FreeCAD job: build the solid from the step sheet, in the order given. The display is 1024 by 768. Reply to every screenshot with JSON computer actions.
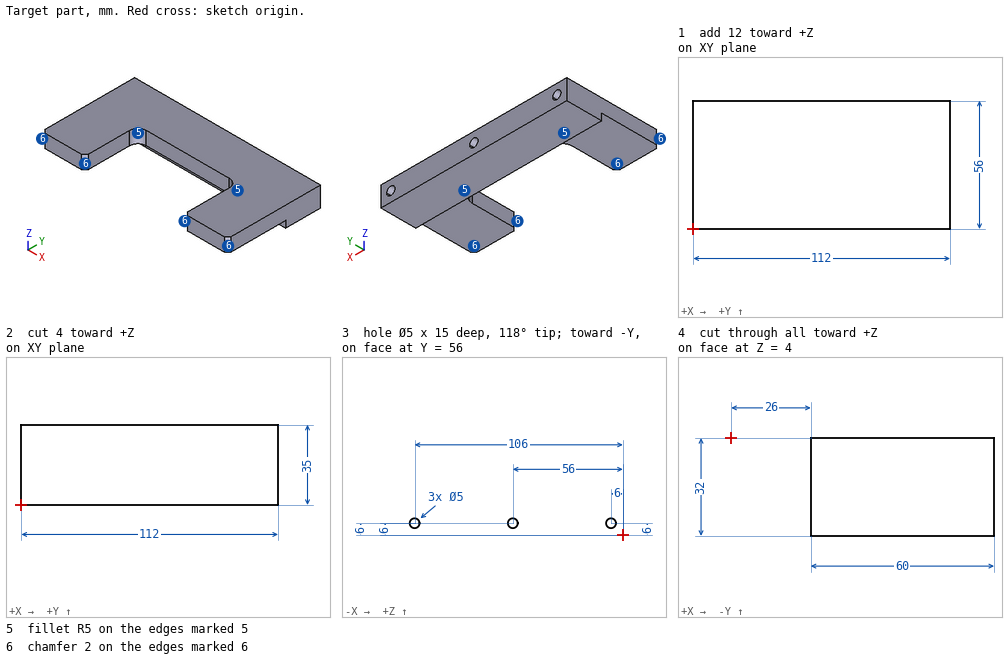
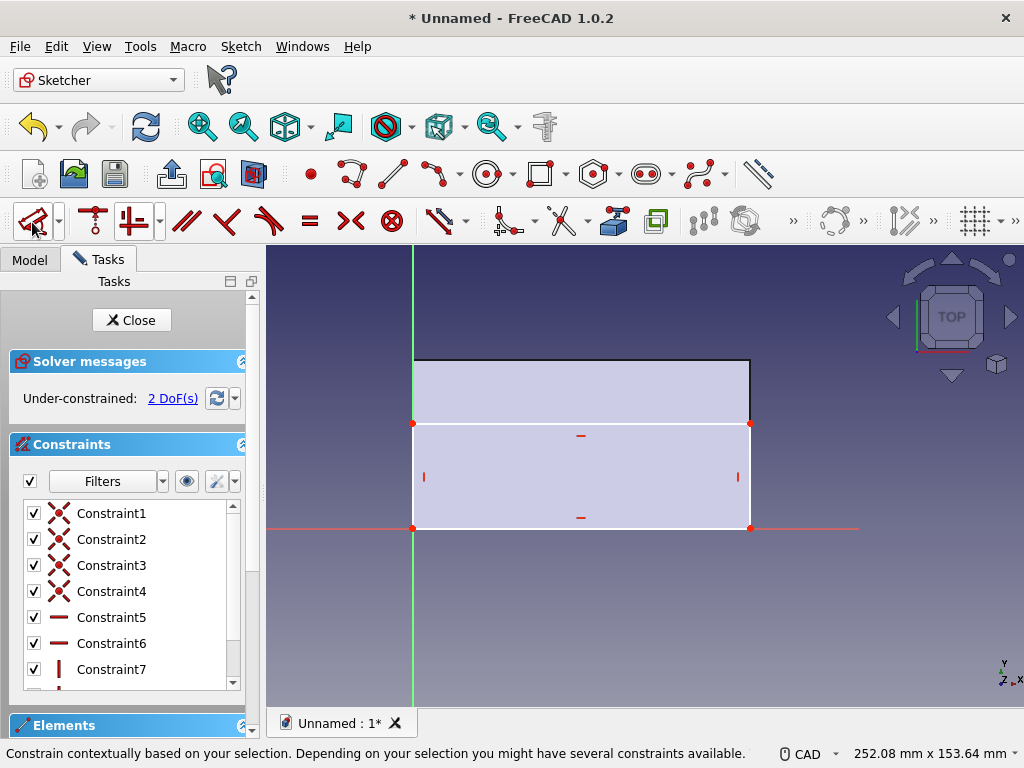
{"action": "left_click", "coordinate": [750, 497]}
{"action": "left_click", "coordinate": [784, 476]}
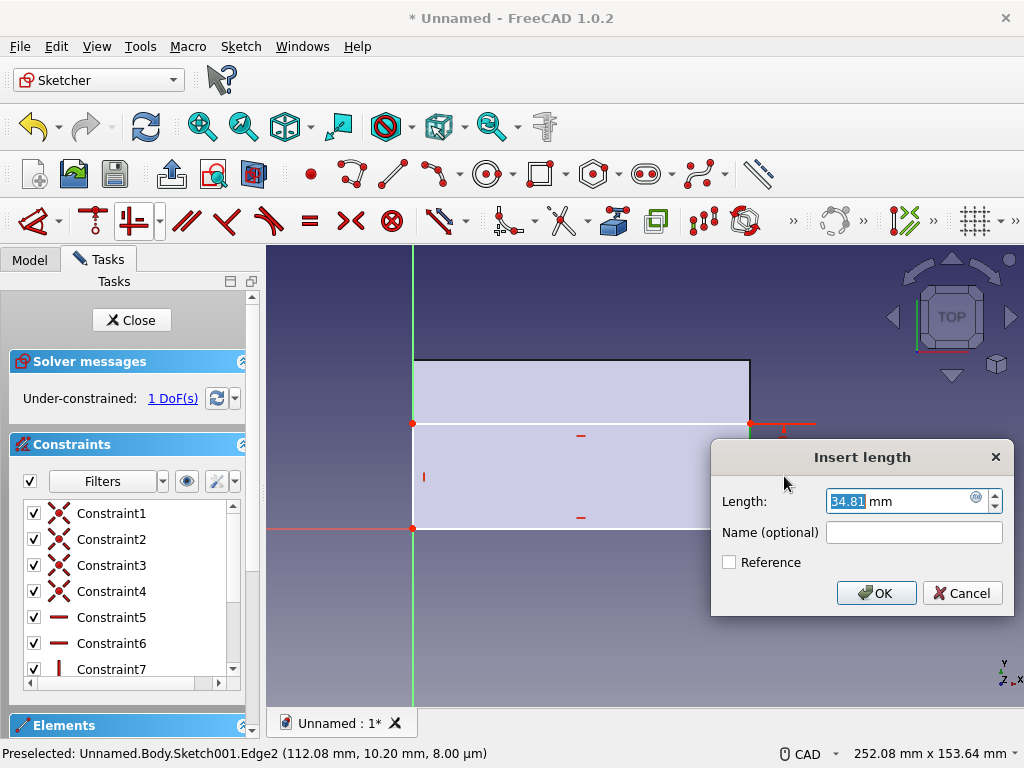
{"action": "type", "text": "35"}
{"action": "key", "text": "Return"}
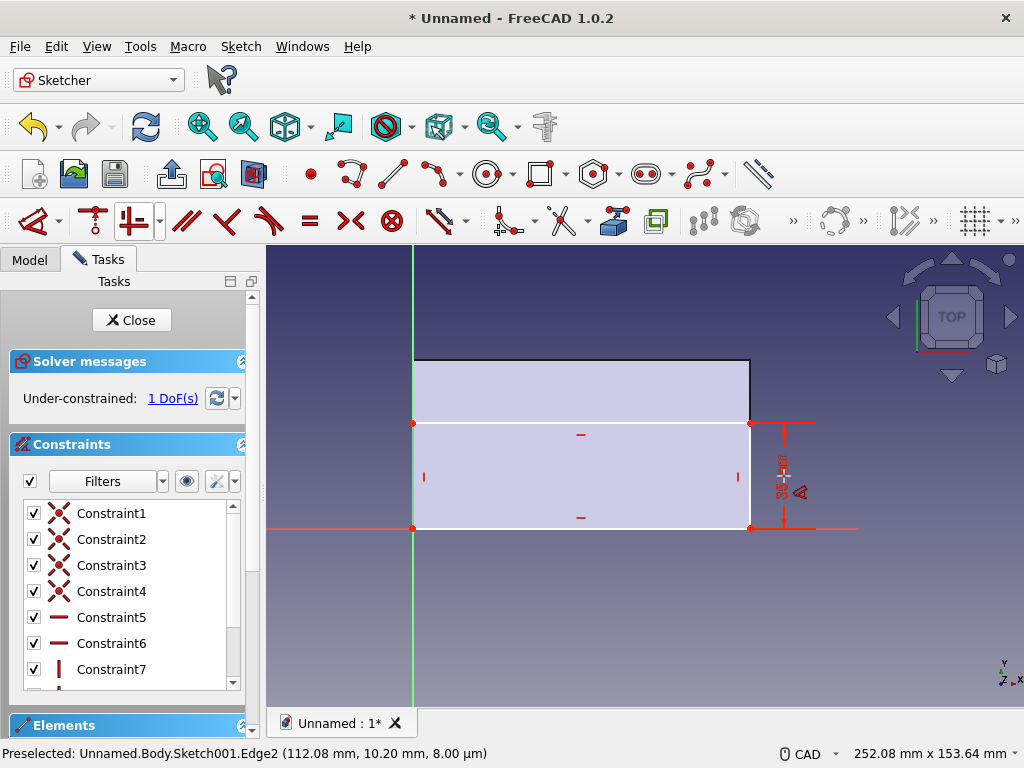
{"action": "left_click", "coordinate": [514, 529]}
{"action": "left_click", "coordinate": [581, 563]}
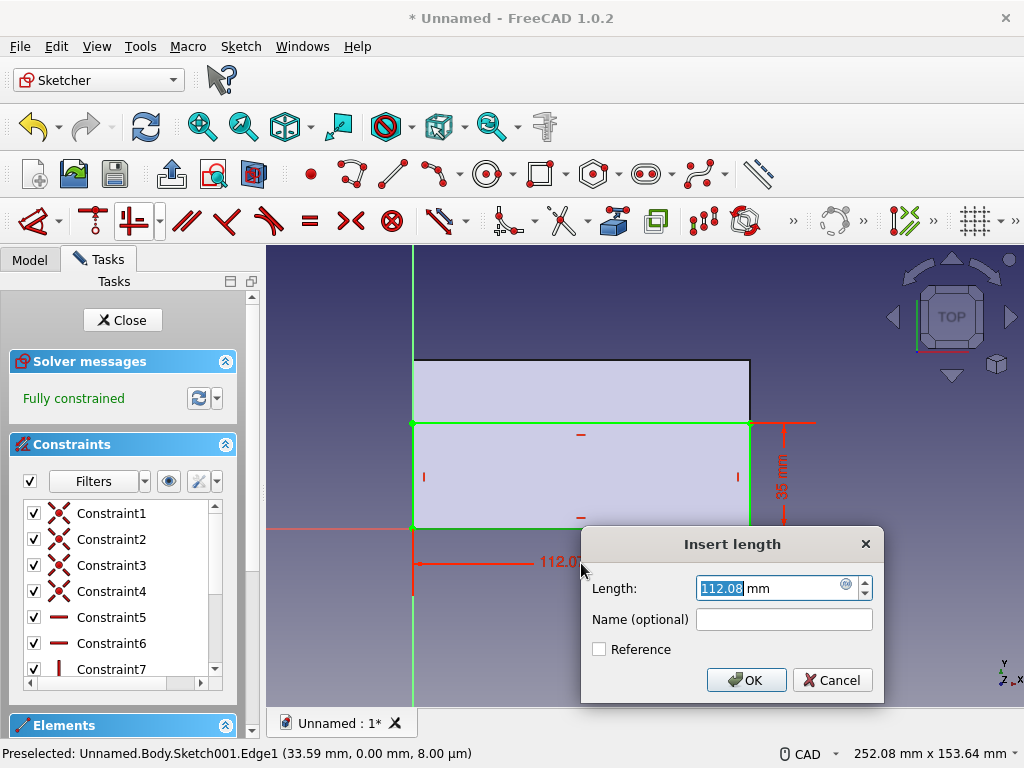
{"action": "type", "text": "112"}
{"action": "key", "text": "Return"}
{"action": "key", "text": "Escape"}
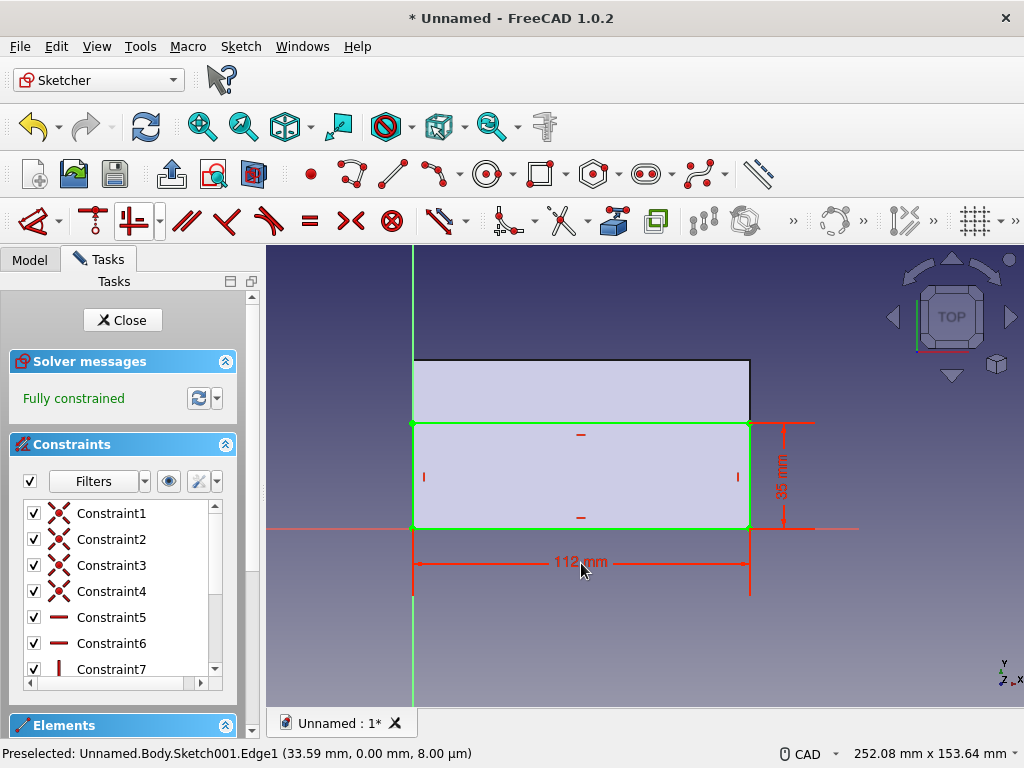
{"action": "left_click", "coordinate": [123, 320]}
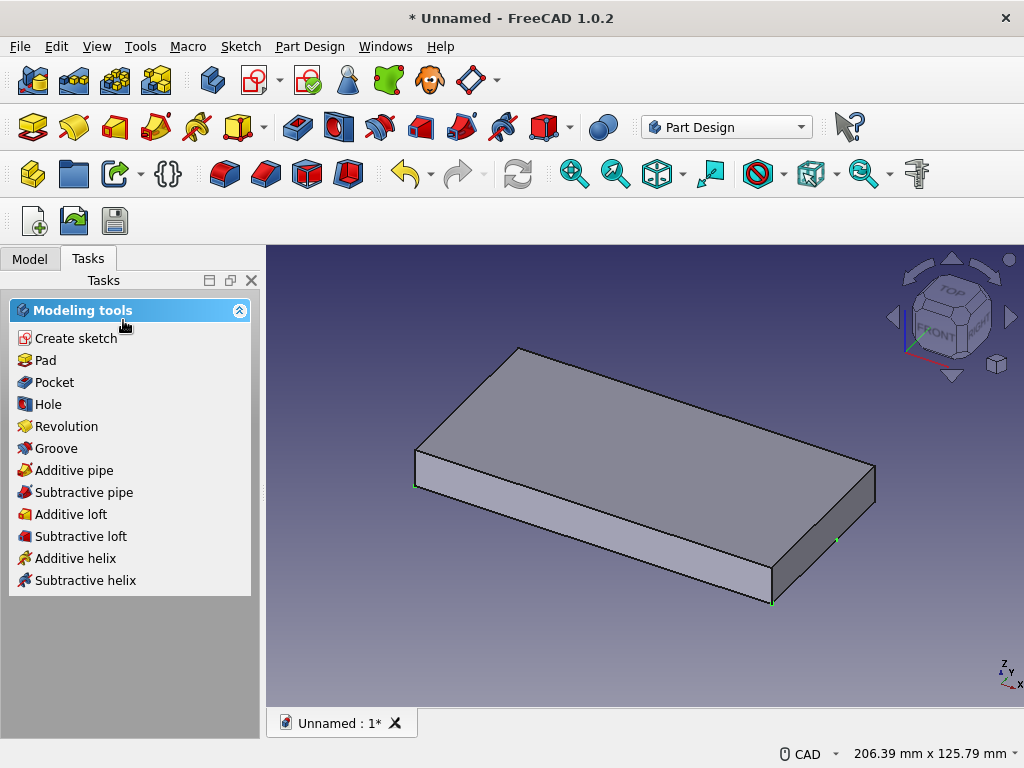
{"action": "left_click", "coordinate": [298, 128]}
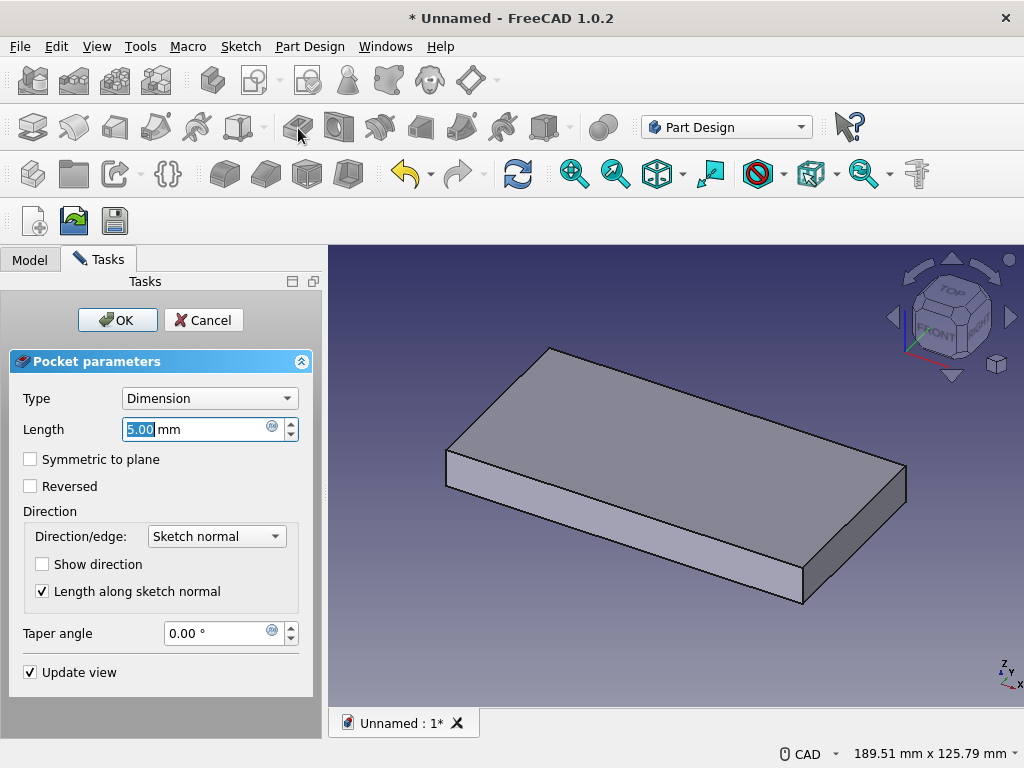
{"action": "type", "text": "4"}
{"action": "key", "text": "Tab"}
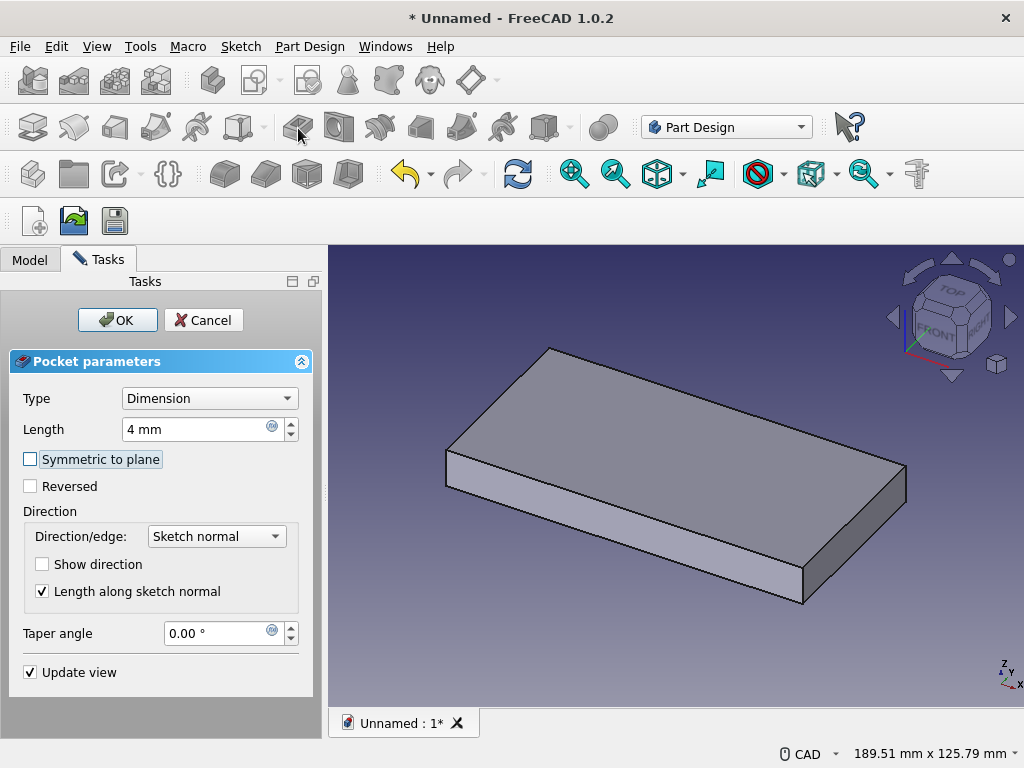
{"action": "left_click", "coordinate": [31, 486]}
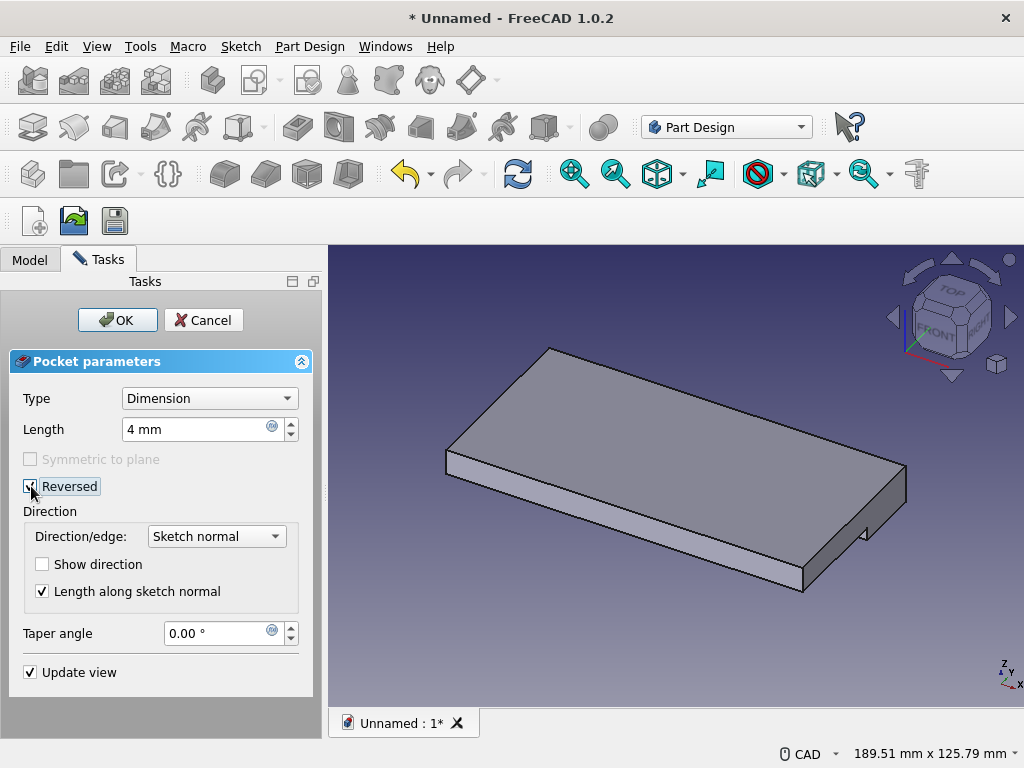
{"action": "left_click", "coordinate": [118, 320]}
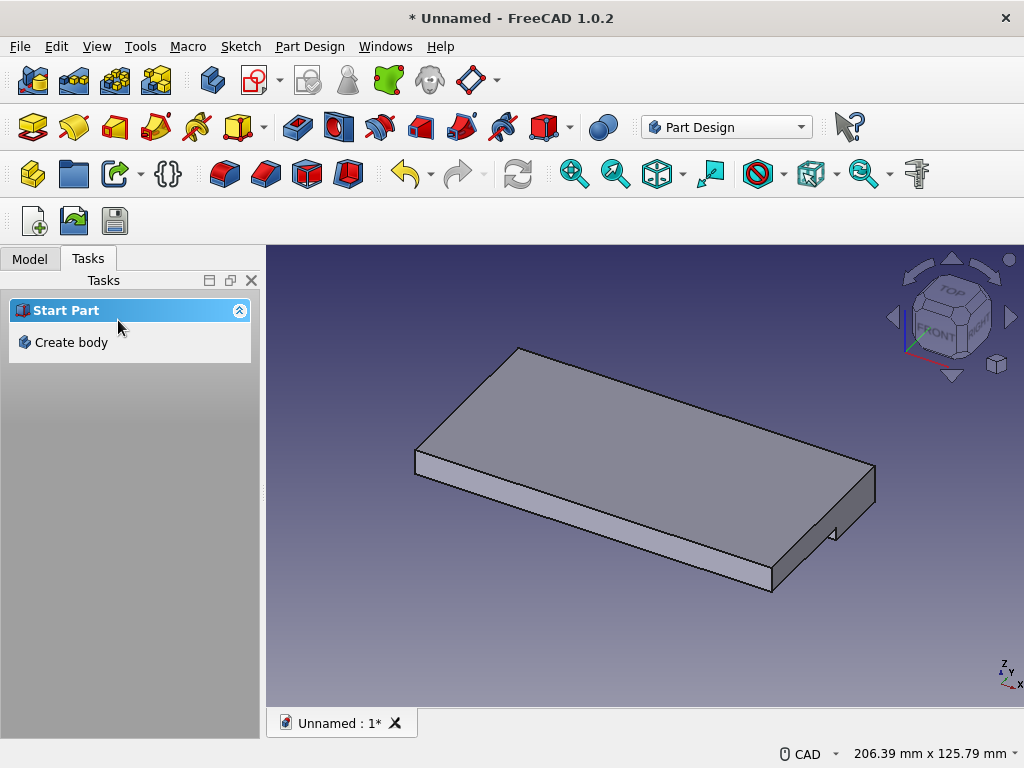
{"action": "key", "text": "4"}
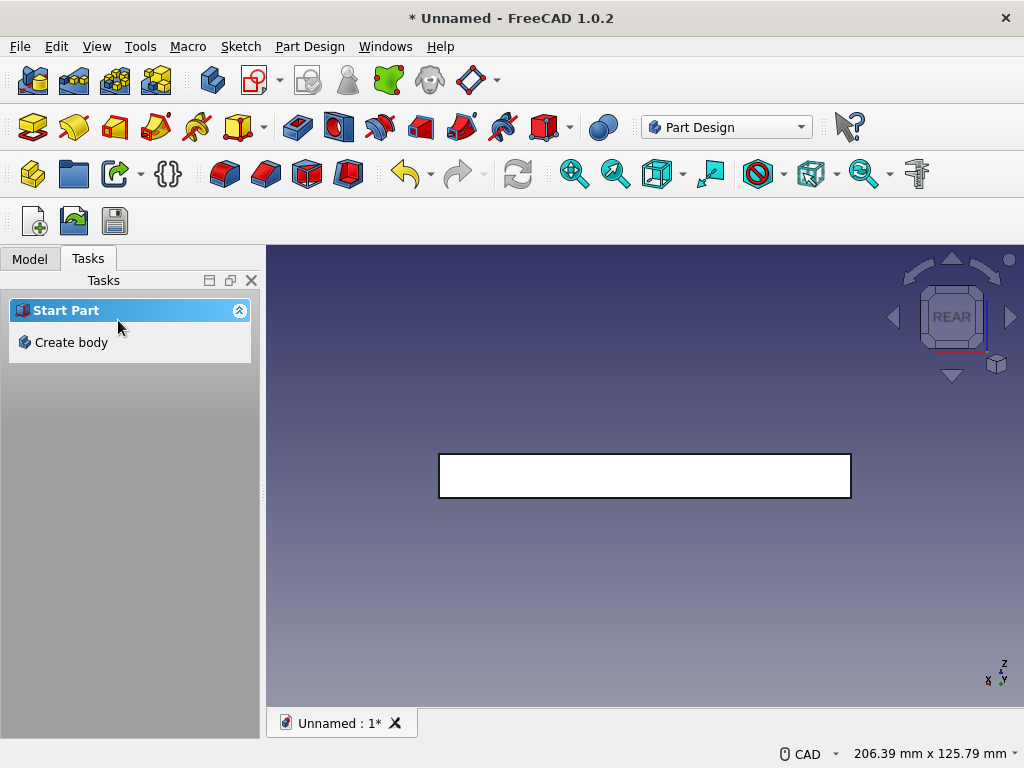
{"action": "left_click", "coordinate": [469, 475]}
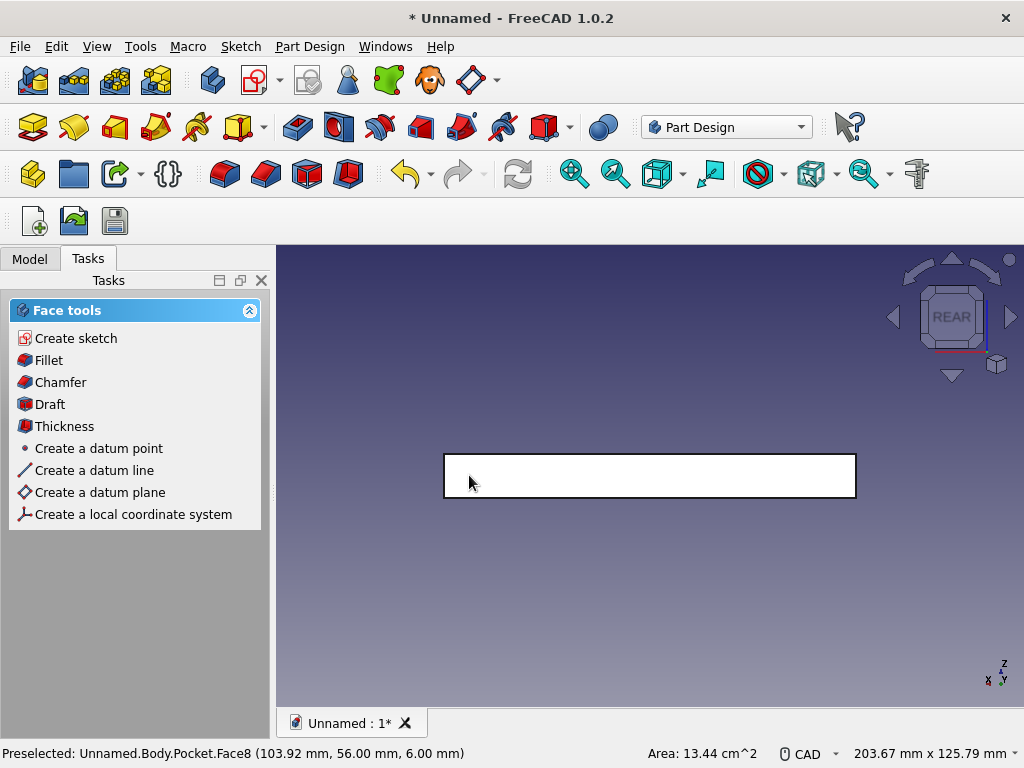
{"action": "left_click", "coordinate": [254, 80]}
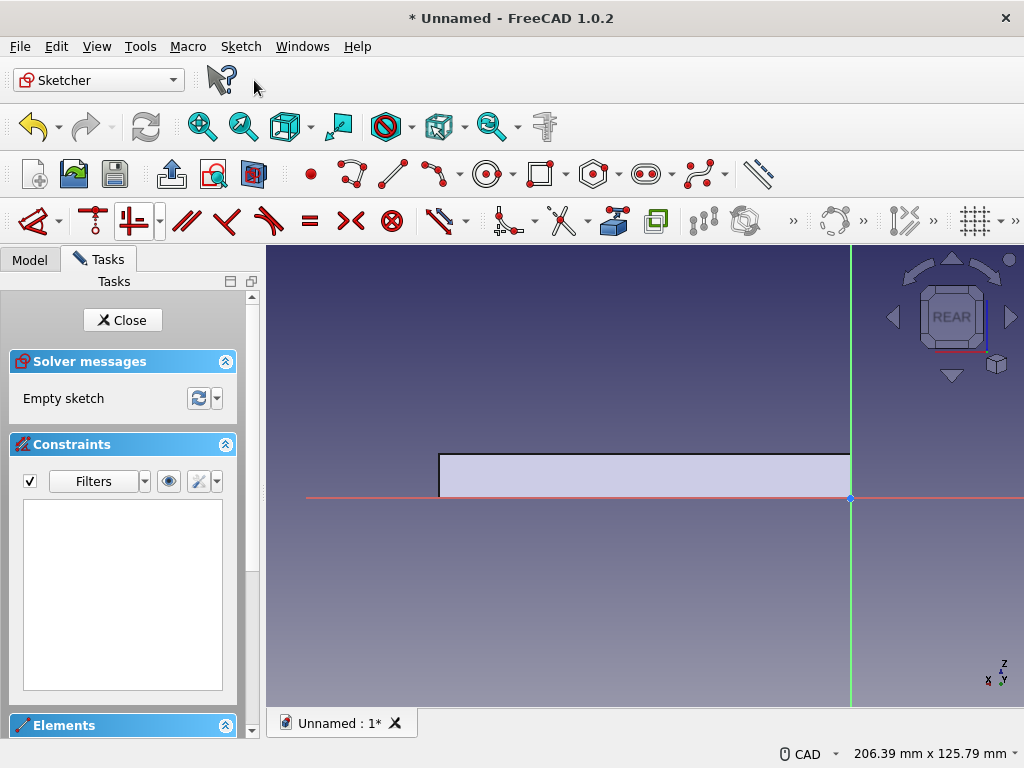
{"action": "scroll", "coordinate": [294, 447], "scroll_direction": "down", "scroll_amount": 1}